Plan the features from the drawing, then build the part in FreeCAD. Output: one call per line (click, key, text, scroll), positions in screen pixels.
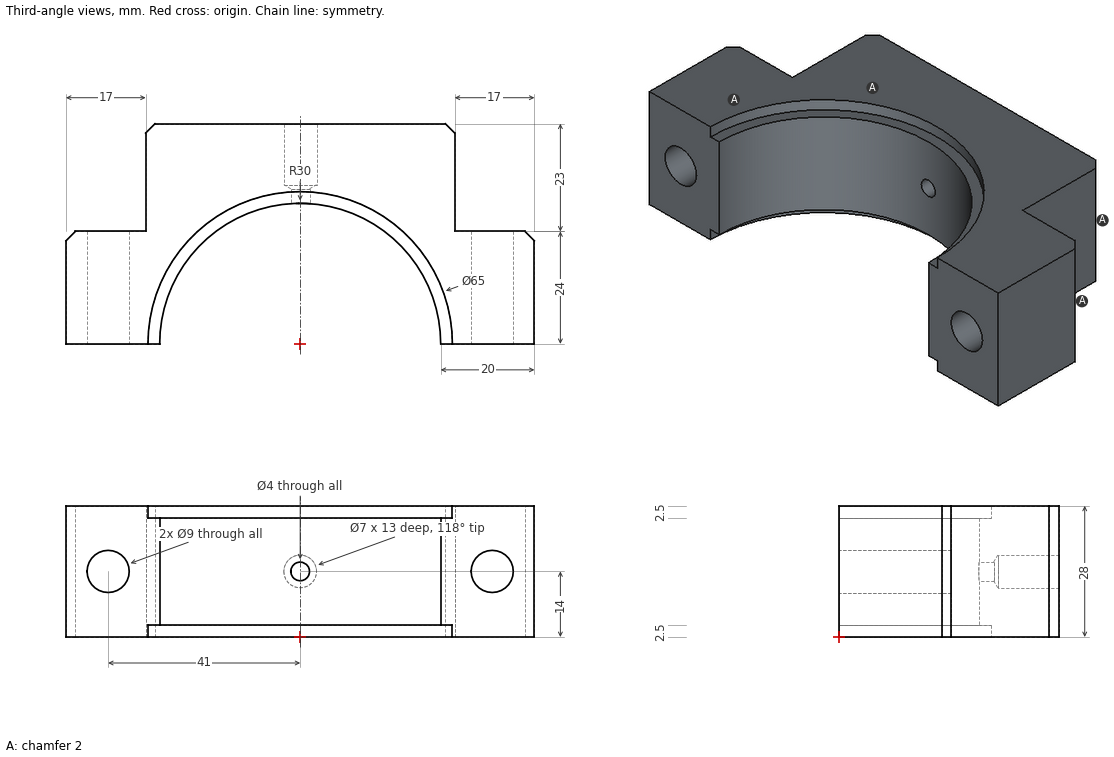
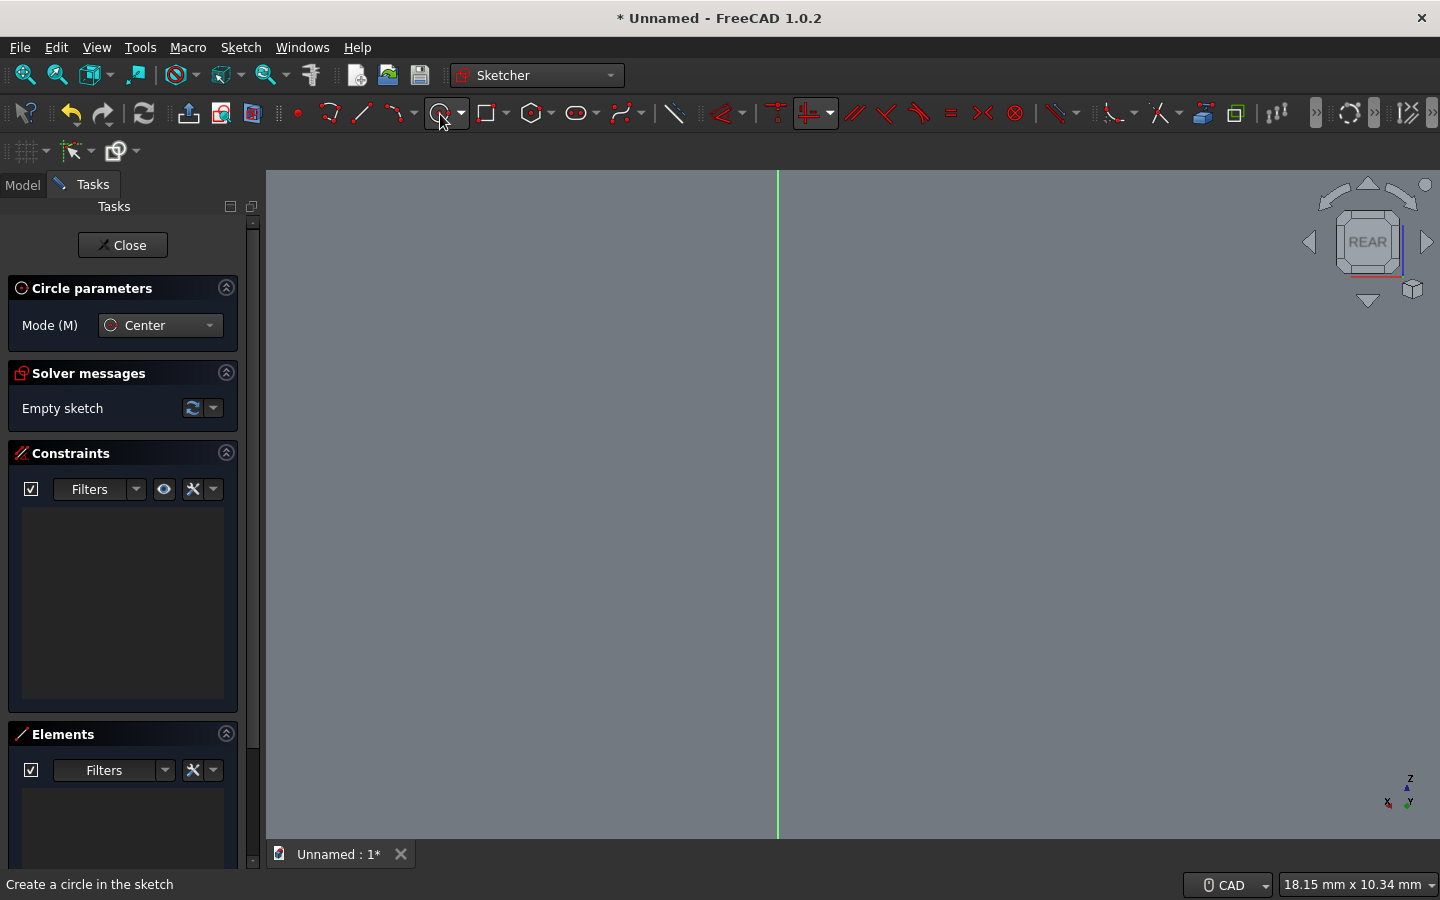
click(778, 504)
click(938, 344)
key(Escape)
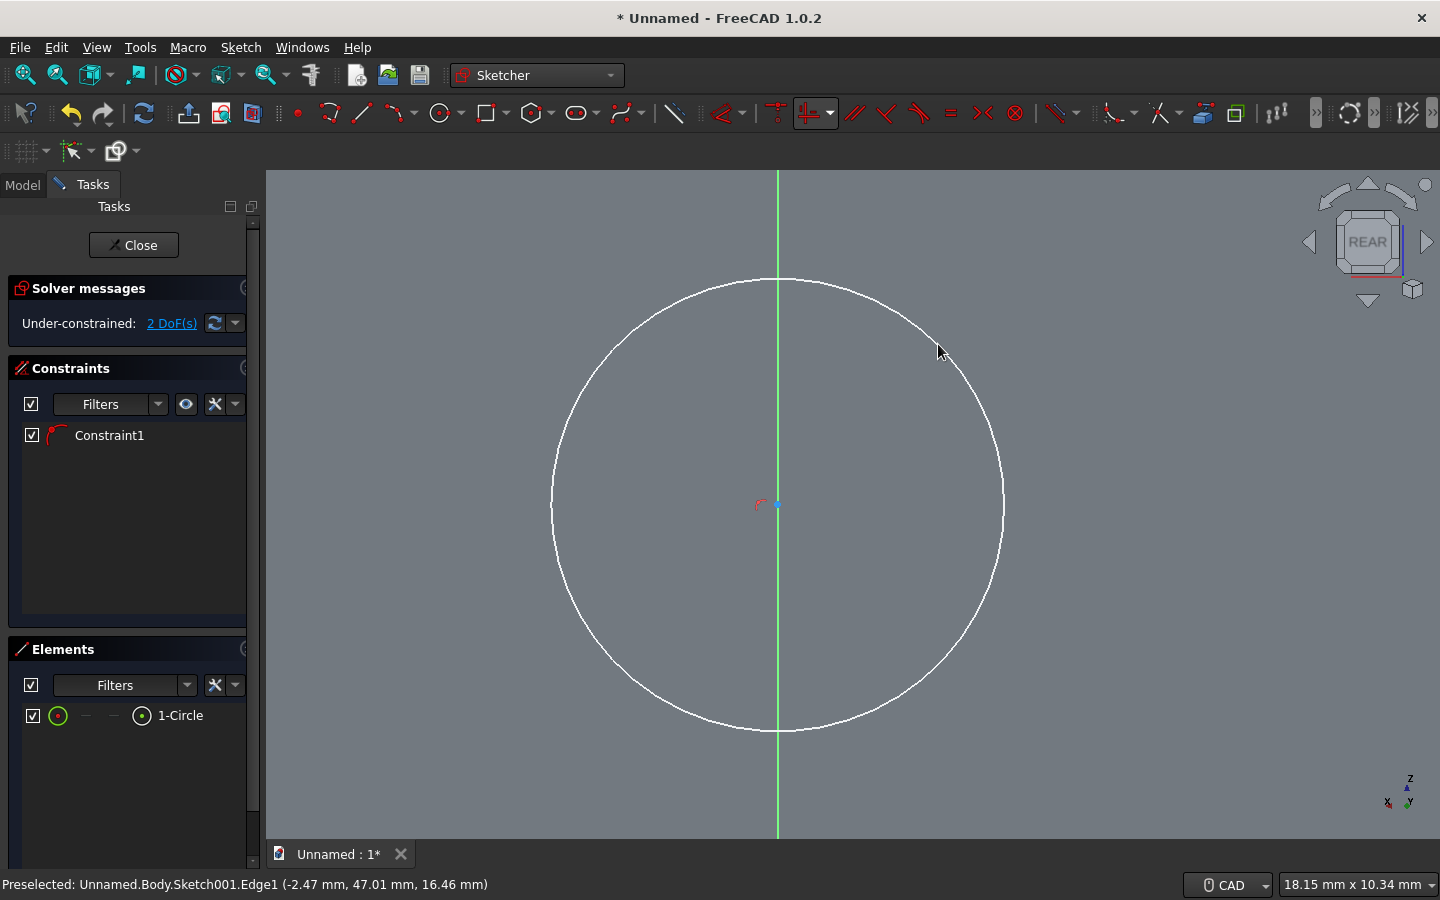
click(722, 114)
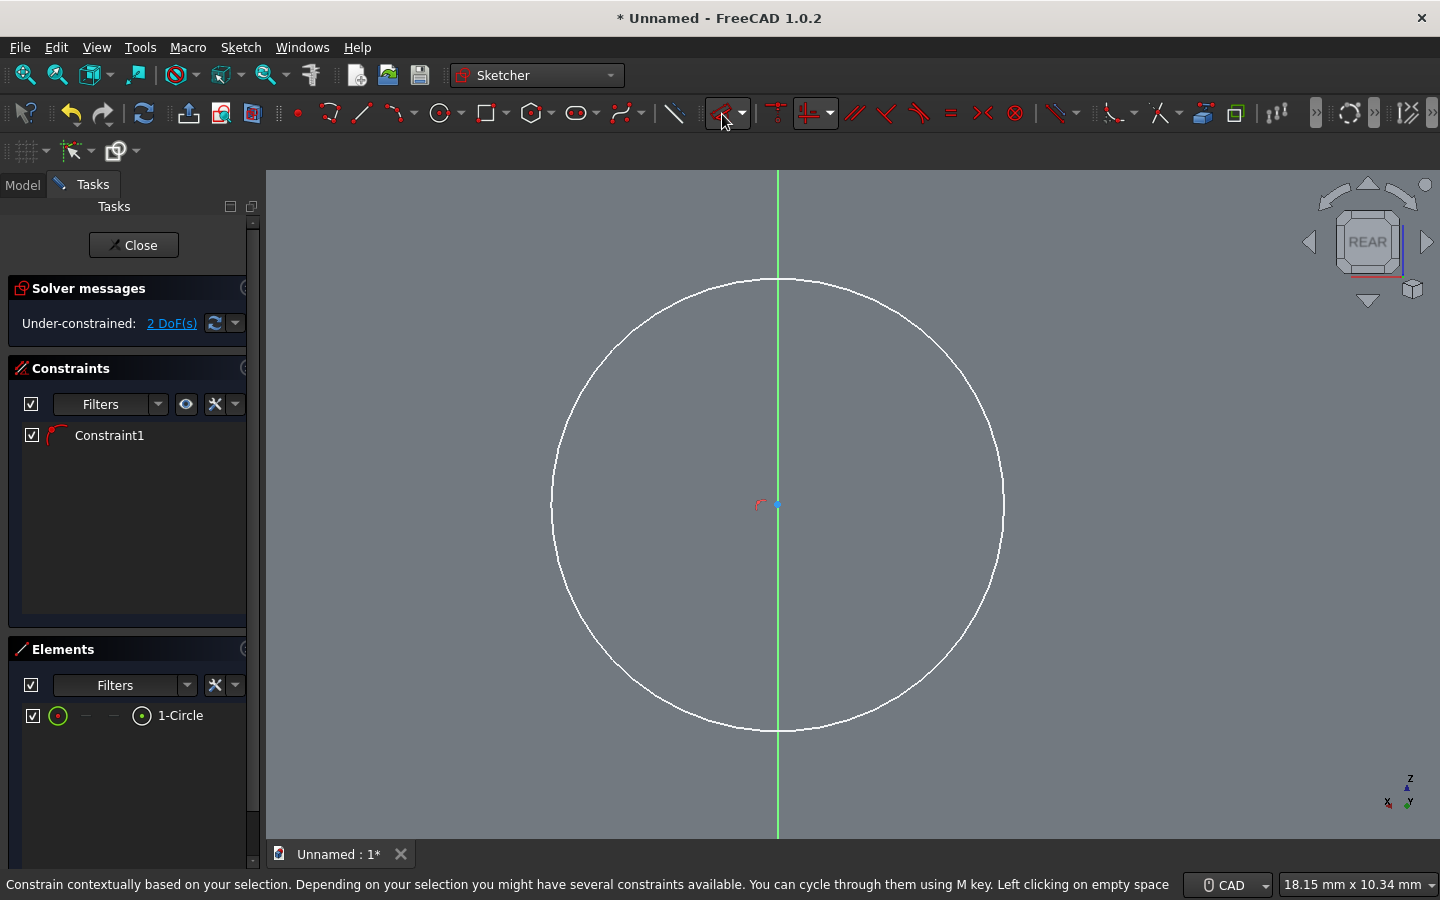
click(937, 344)
click(960, 321)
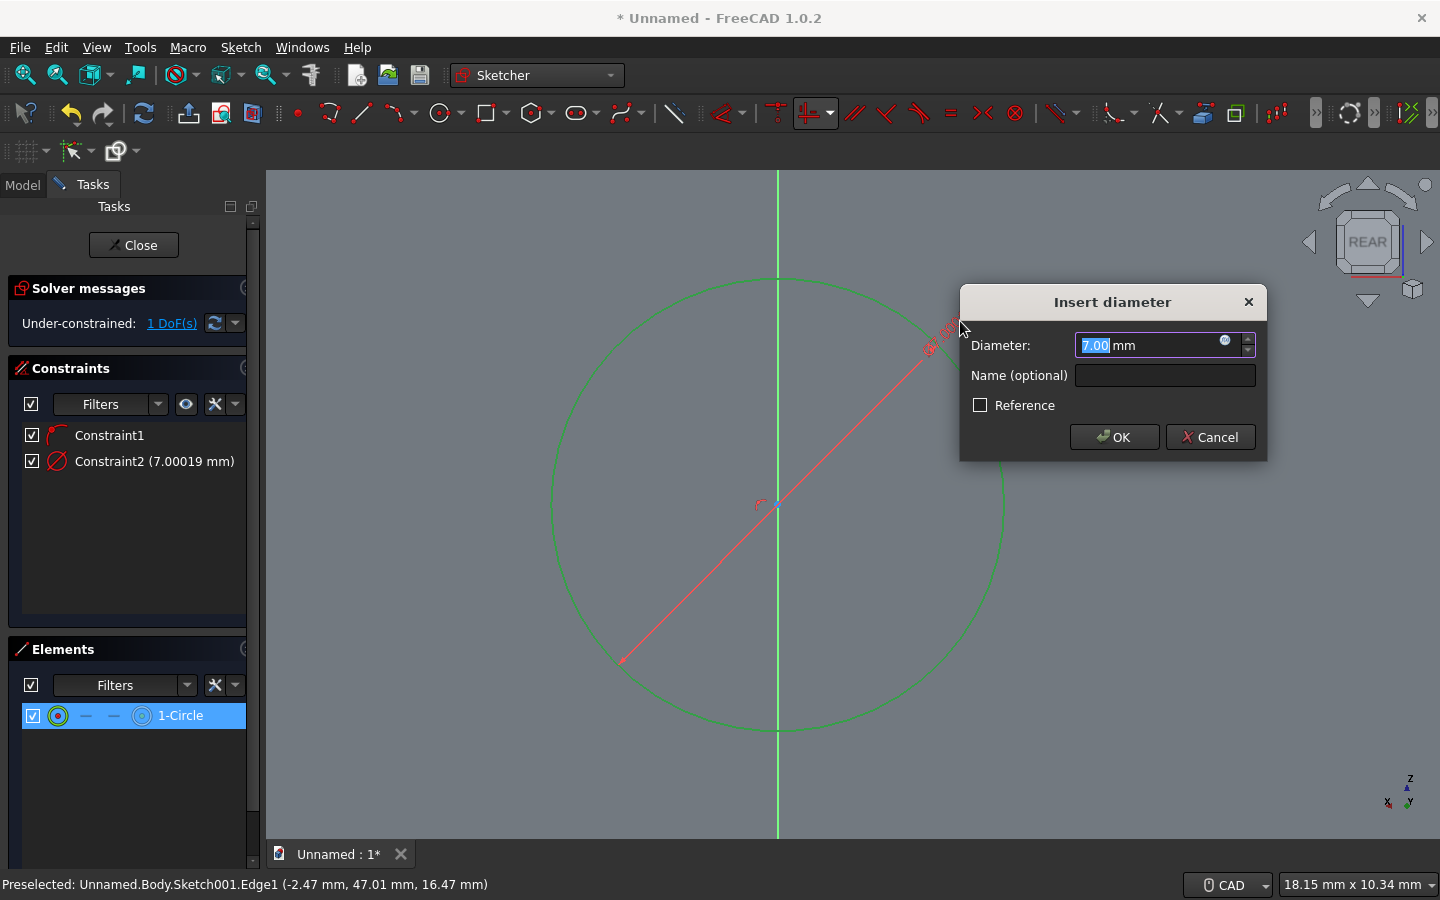
text(7)
key(Return)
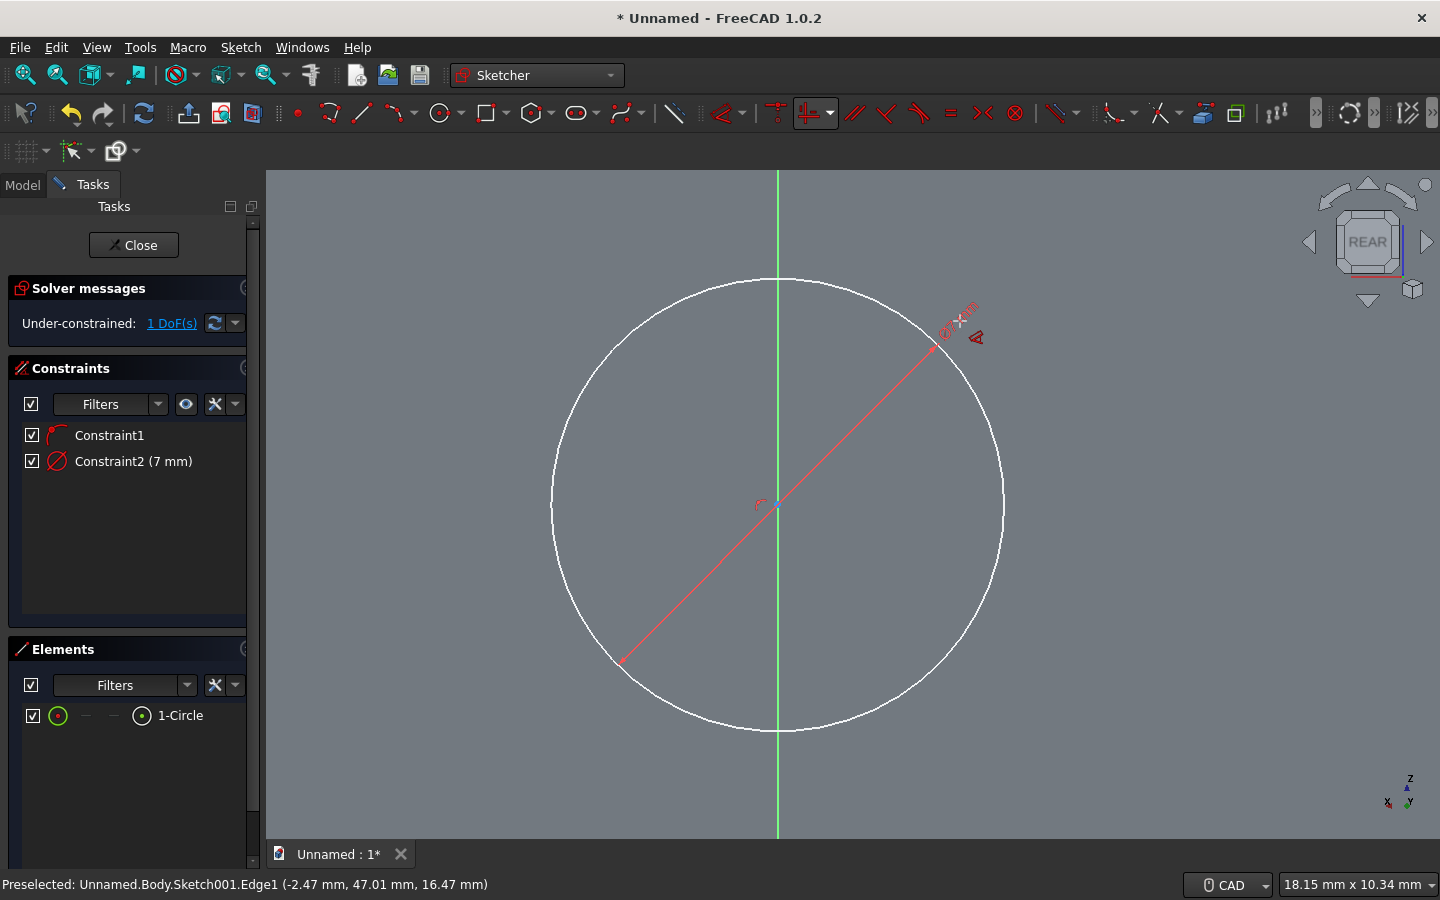
click(778, 505)
click(812, 658)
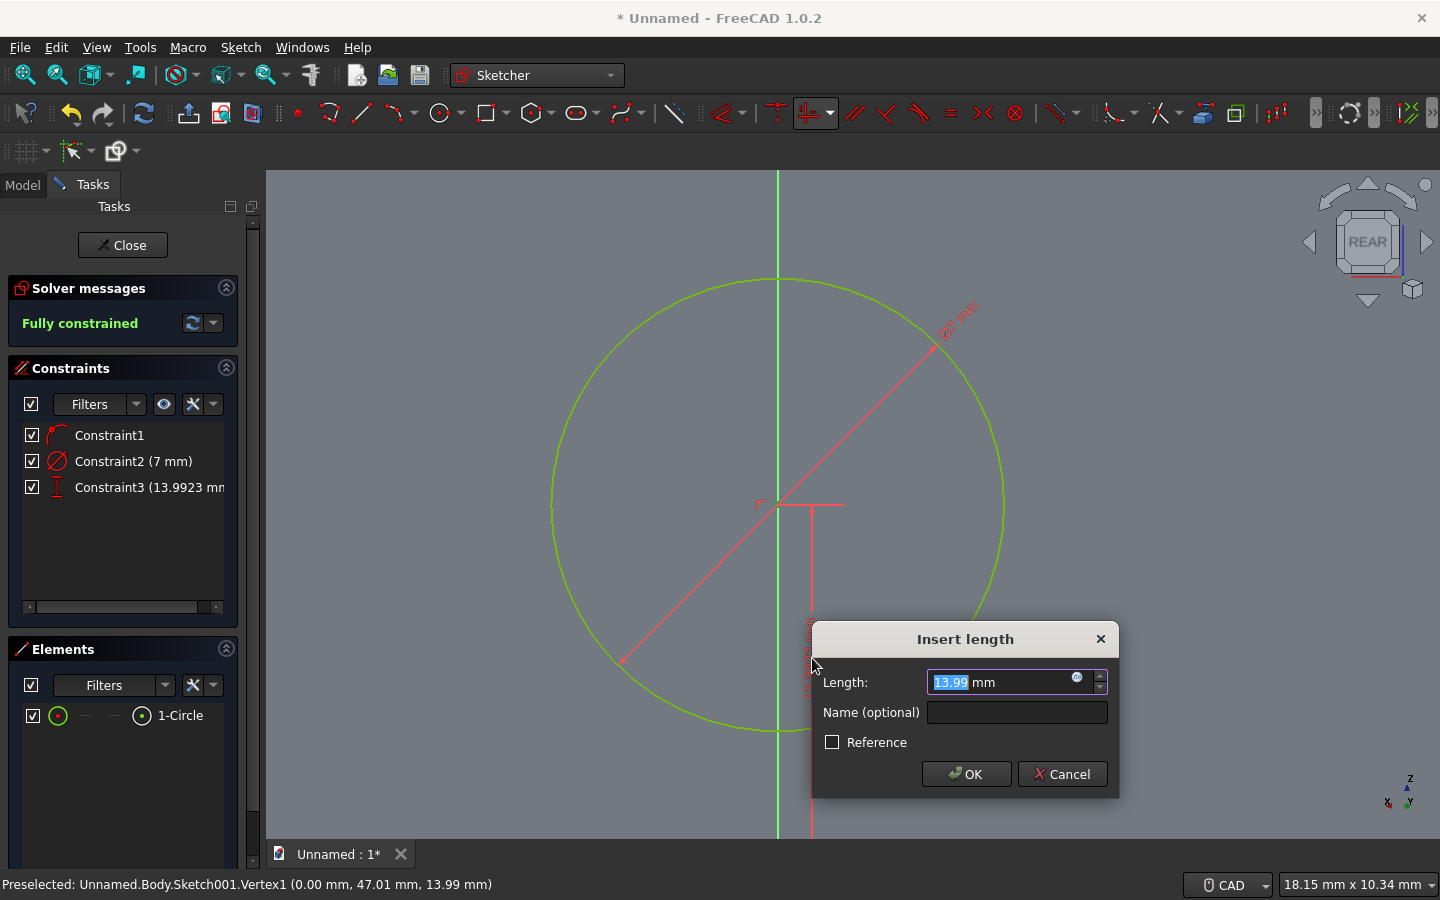
text(14)
key(Return)
key(Escape)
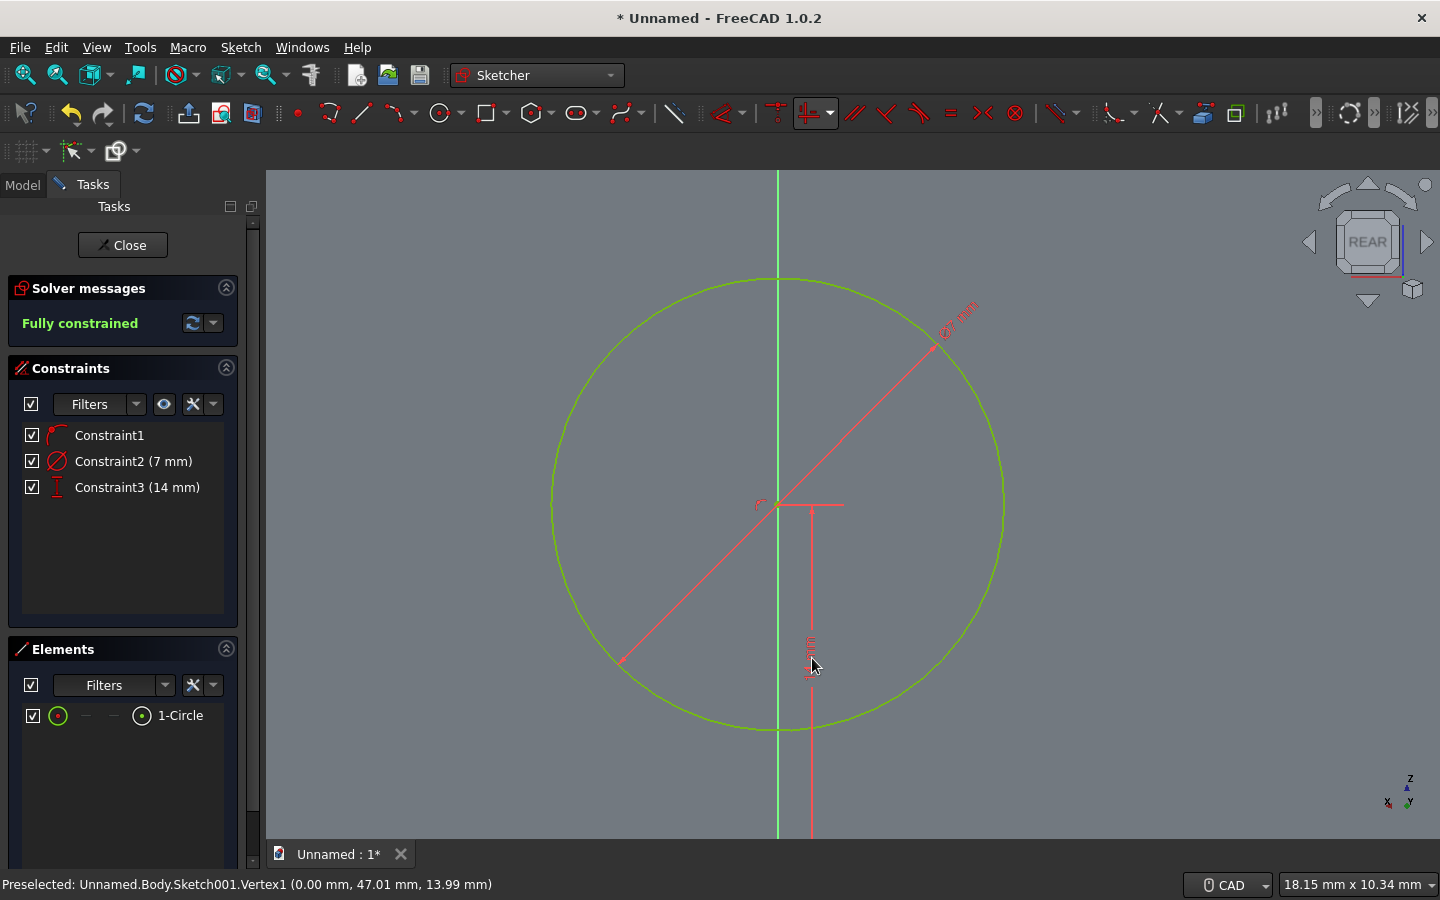
click(123, 245)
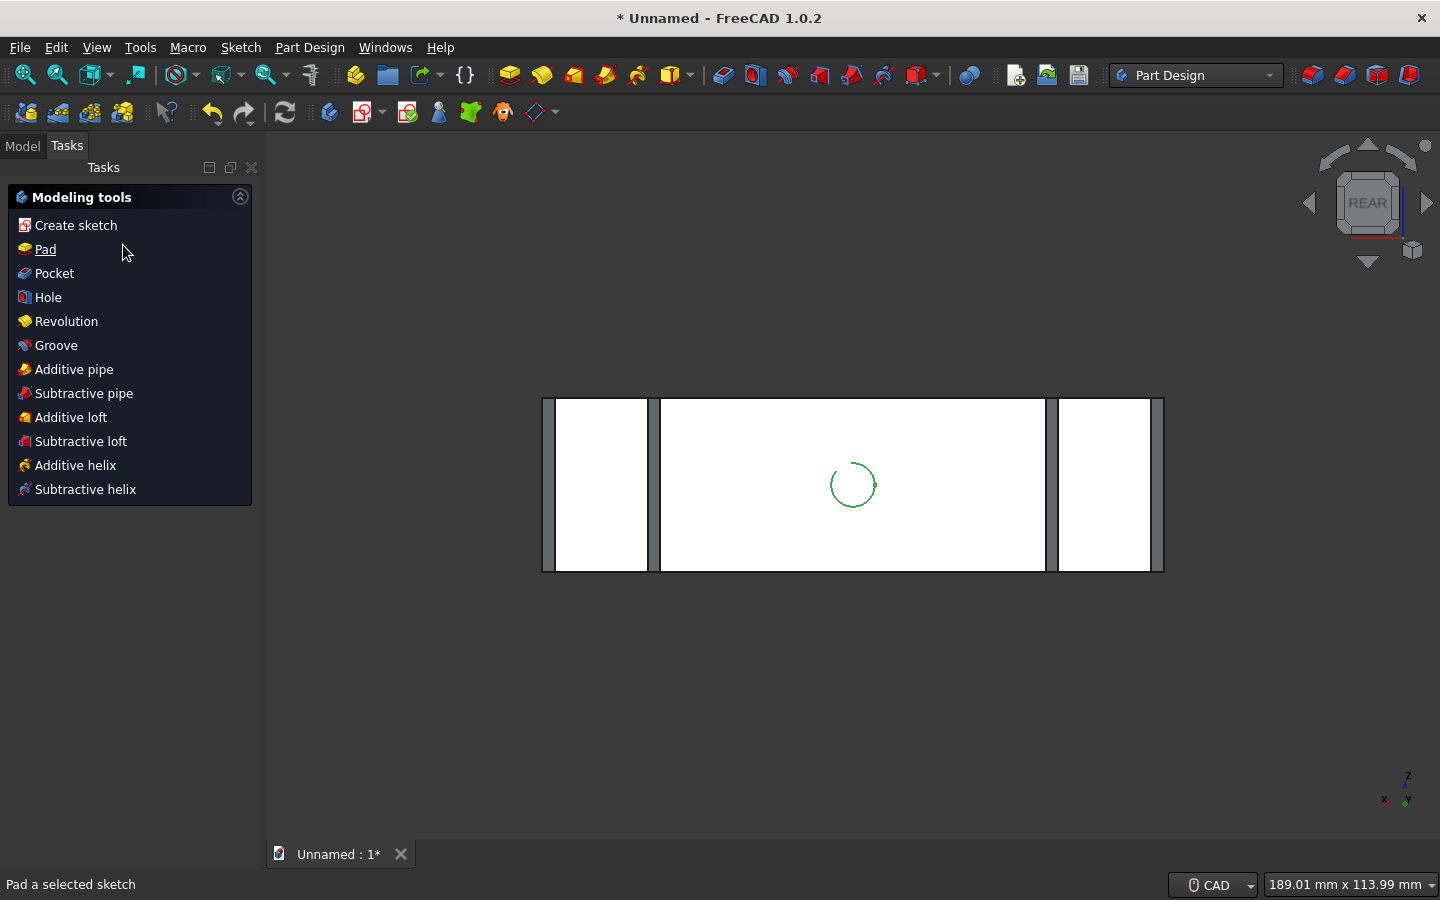
click(756, 76)